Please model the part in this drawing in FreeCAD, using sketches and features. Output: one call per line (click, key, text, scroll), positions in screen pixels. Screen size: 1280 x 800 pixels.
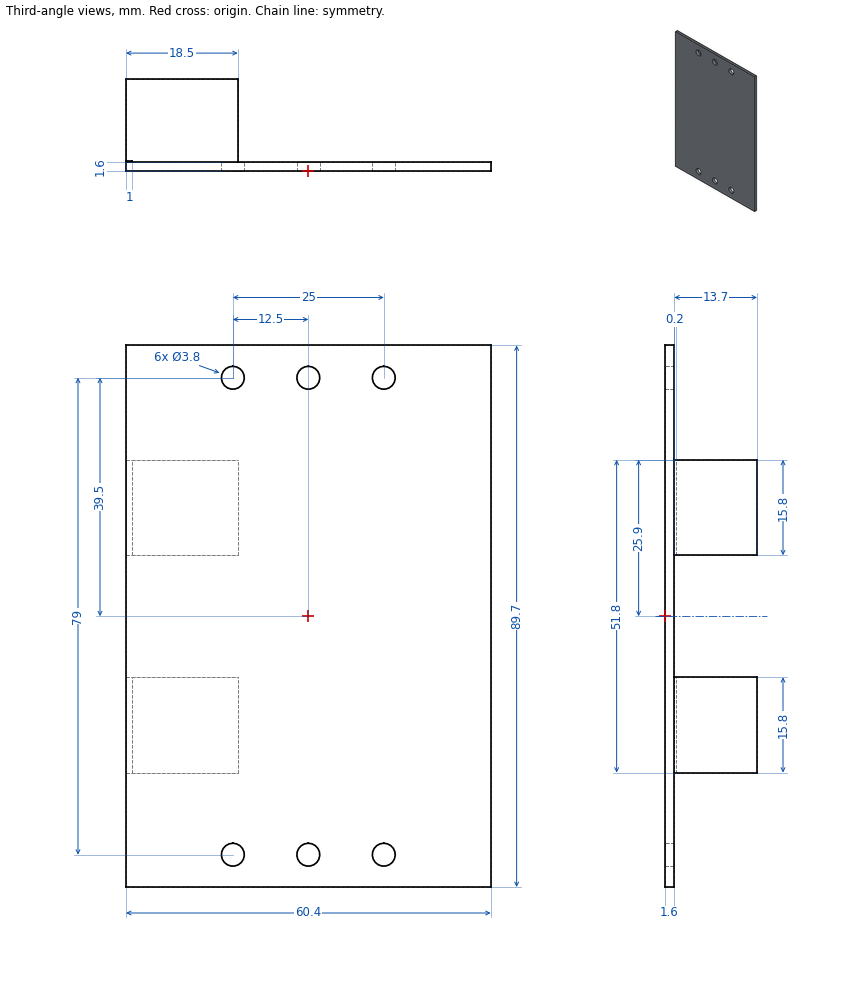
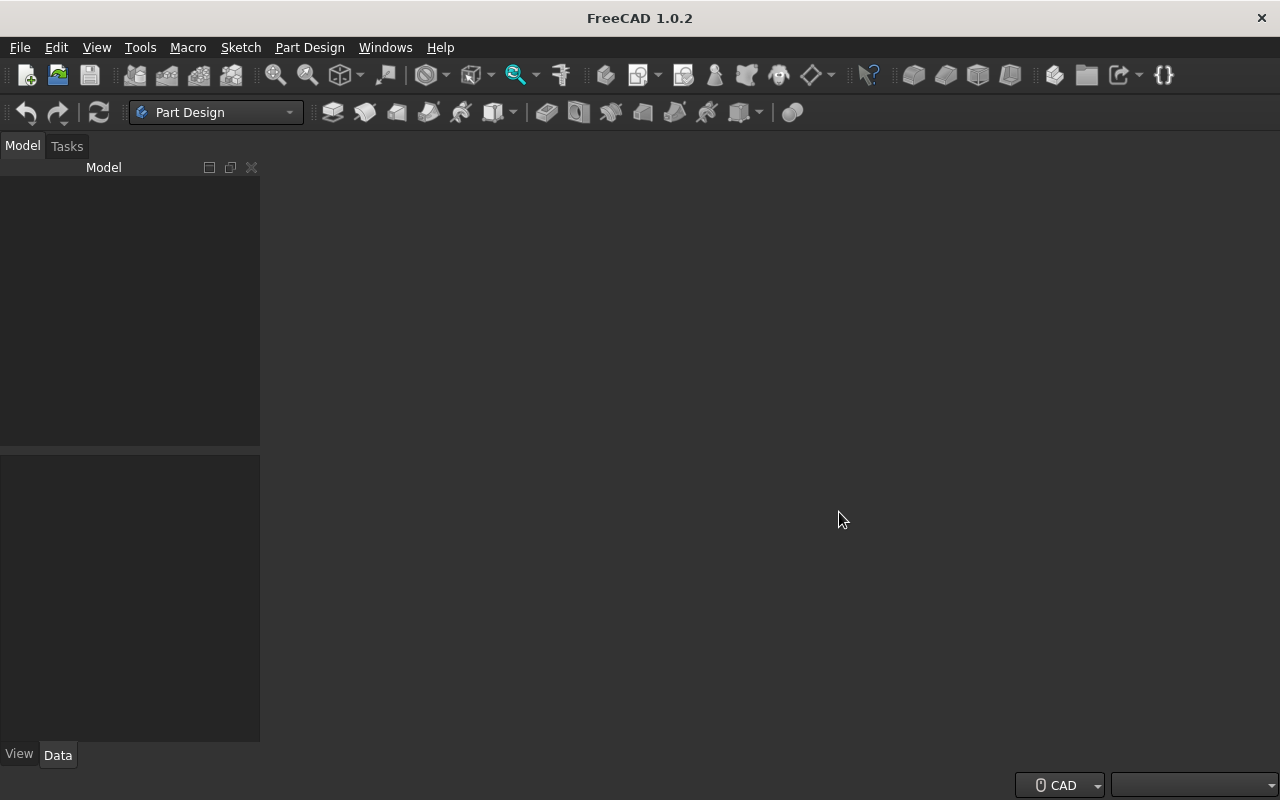
click(26, 76)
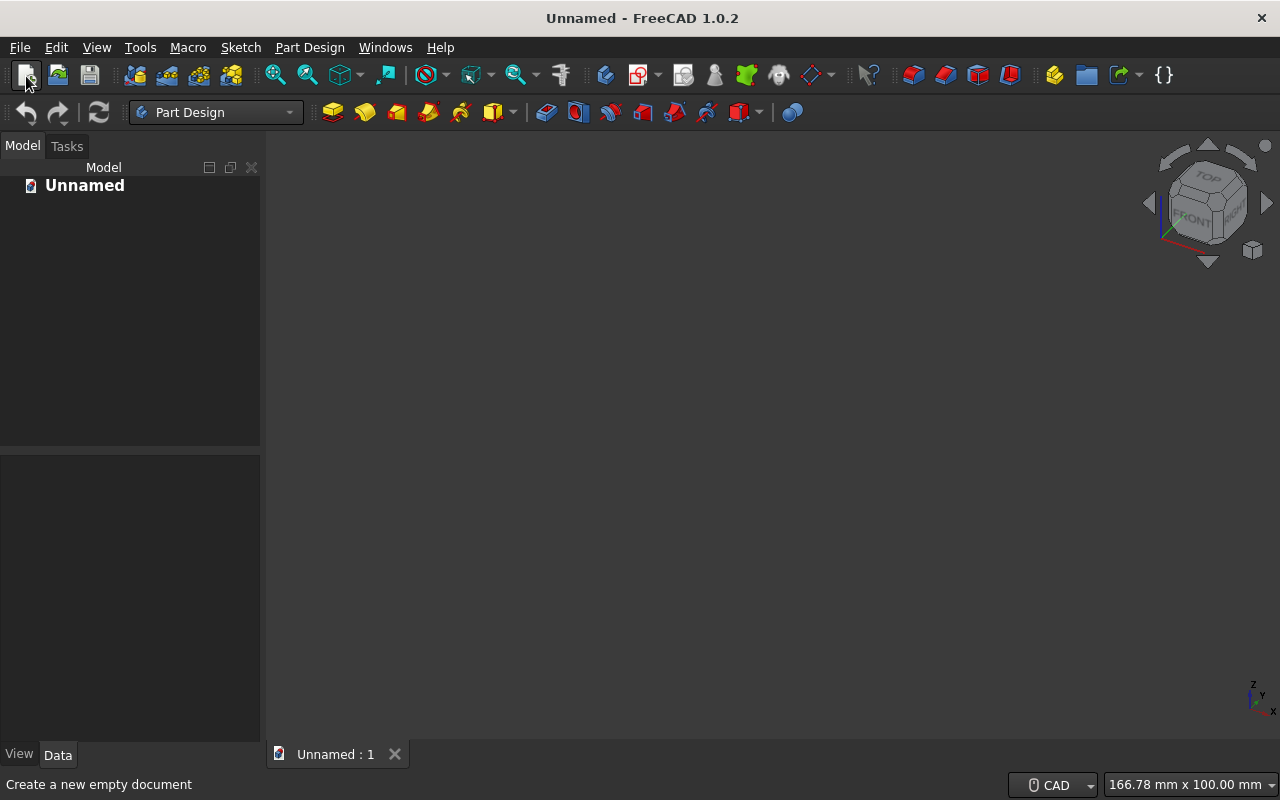
click(638, 76)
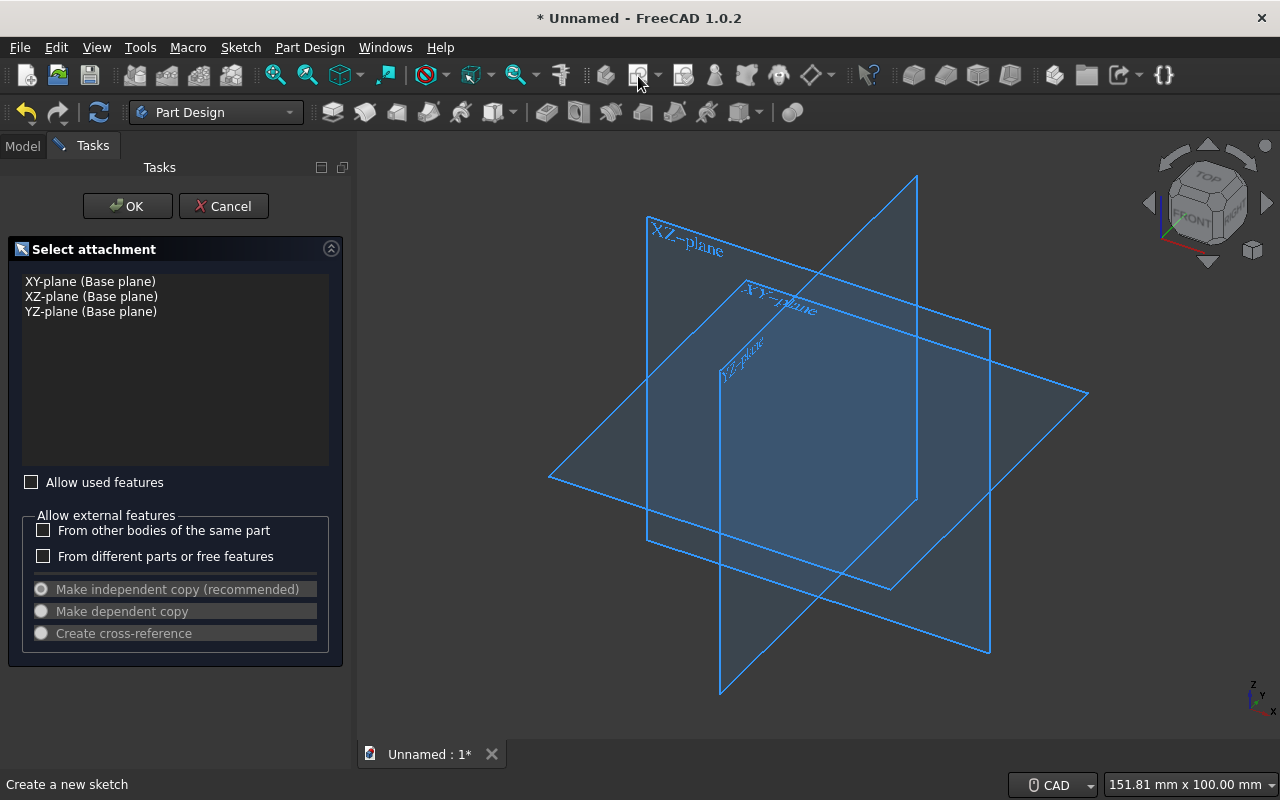
click(82, 296)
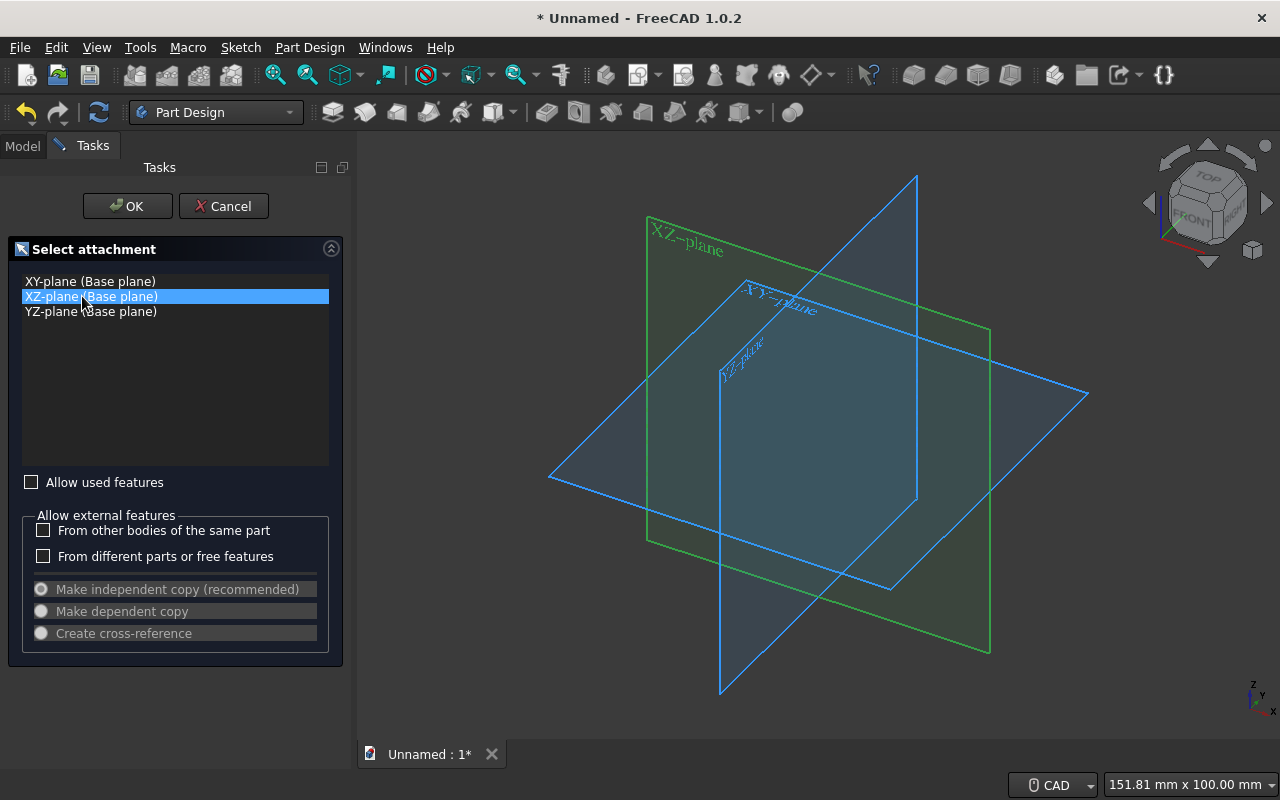
click(128, 206)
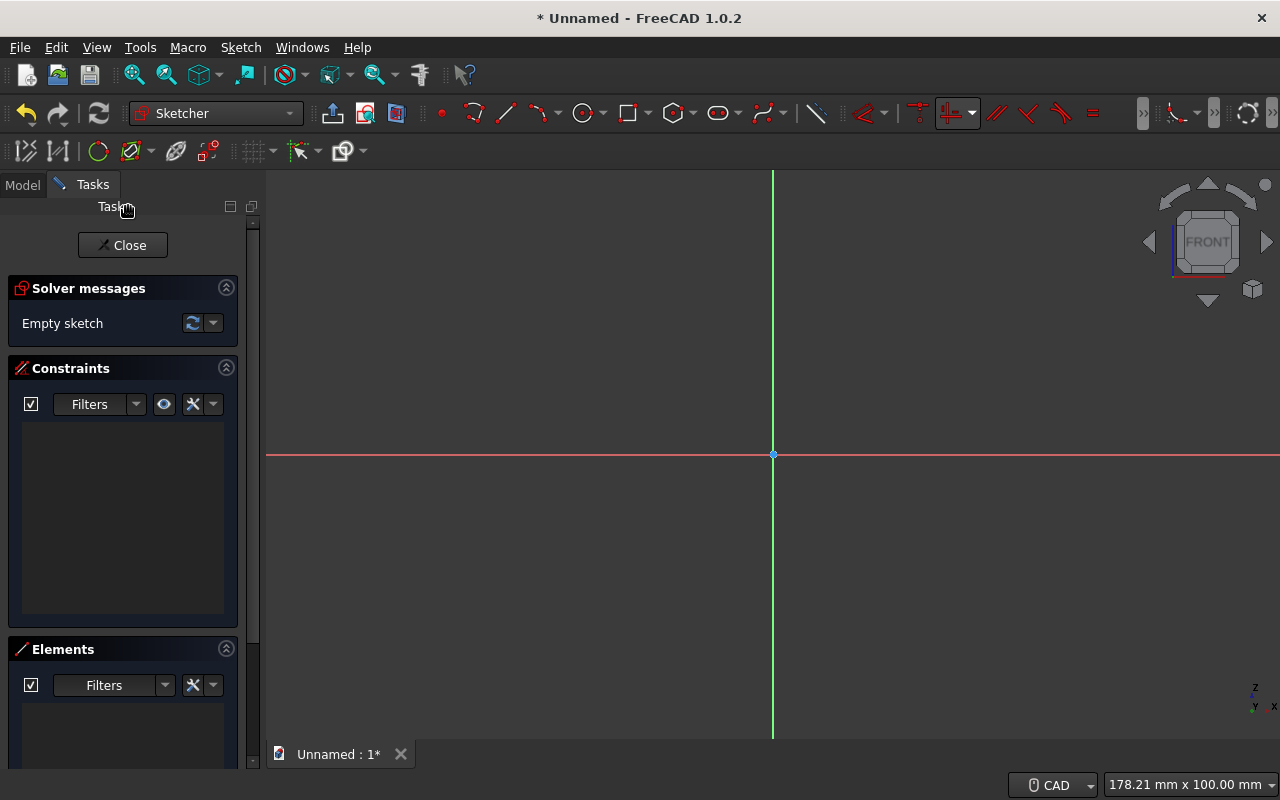
scroll(565, 455, down, 2)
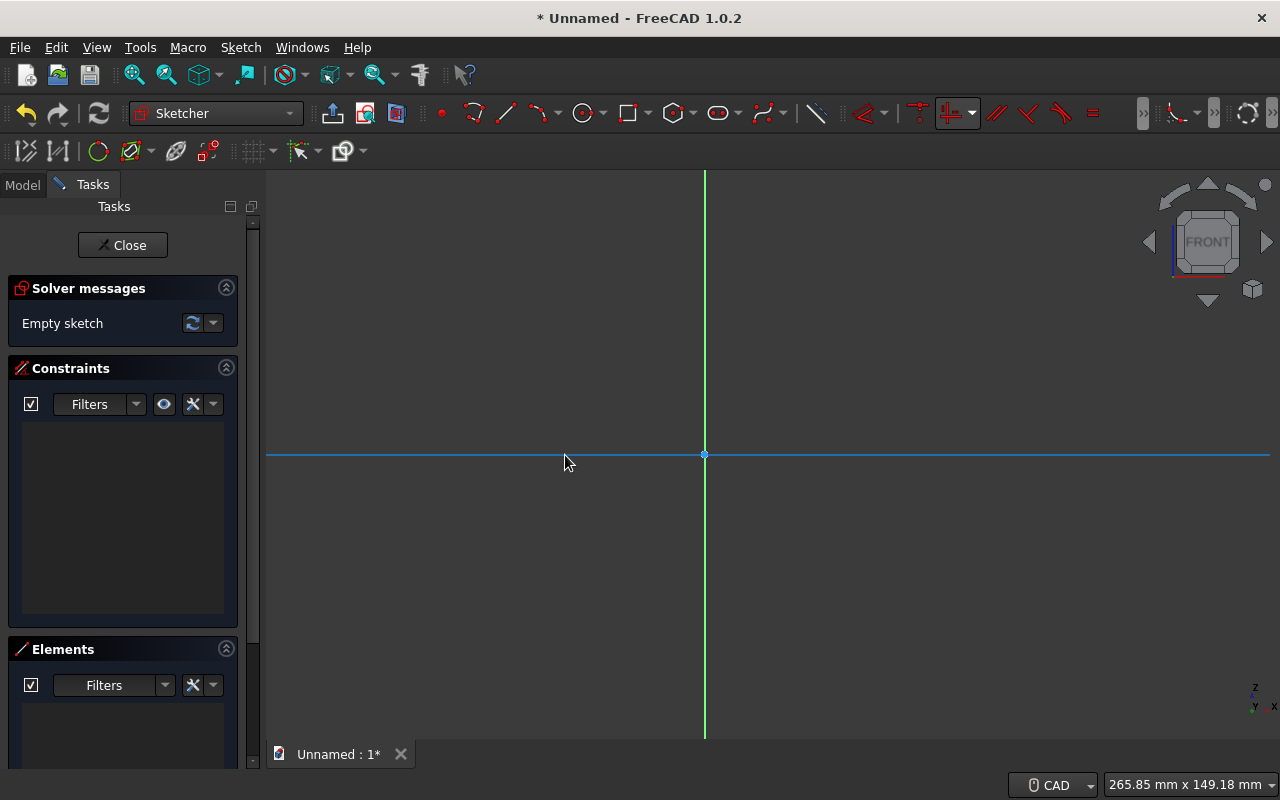
key(g)
key(v)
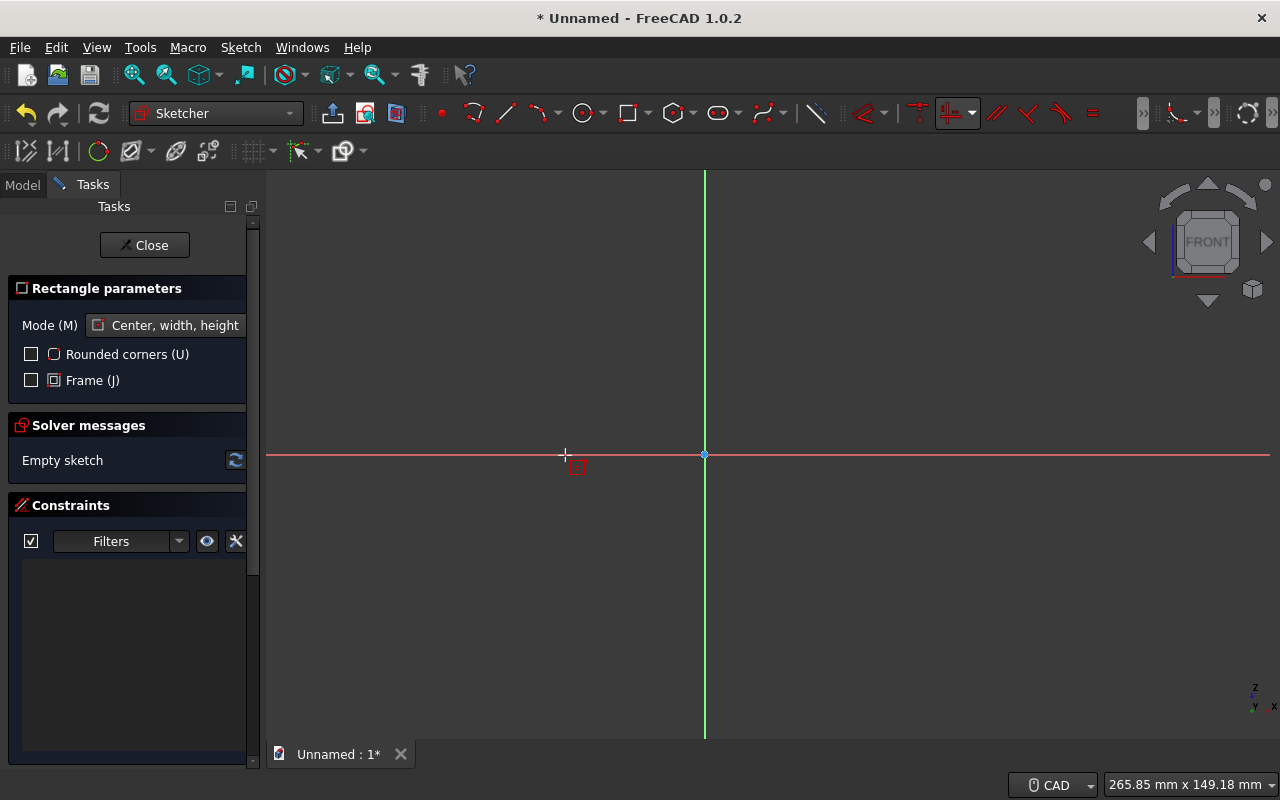
click(705, 455)
move(820, 284)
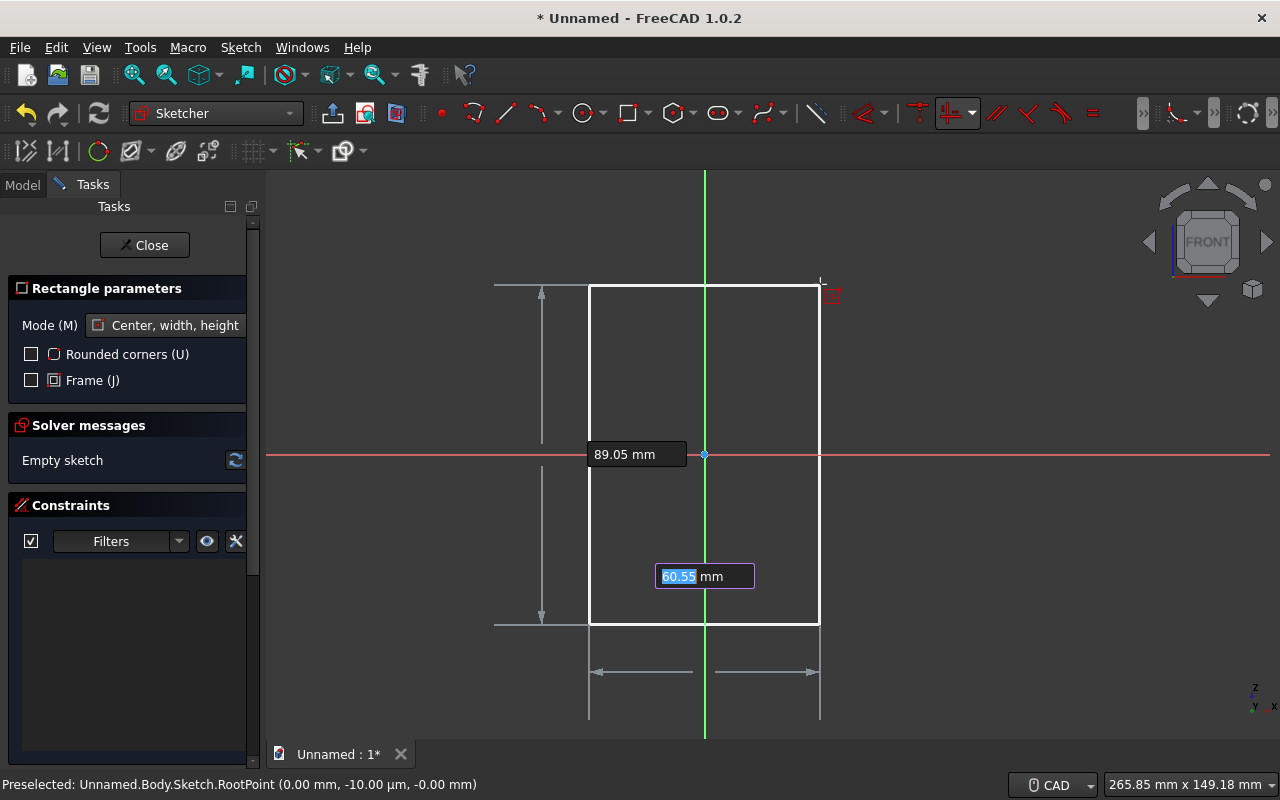
text(60.4)
key(Tab)
text(89.7)
key(Return)
key(Escape)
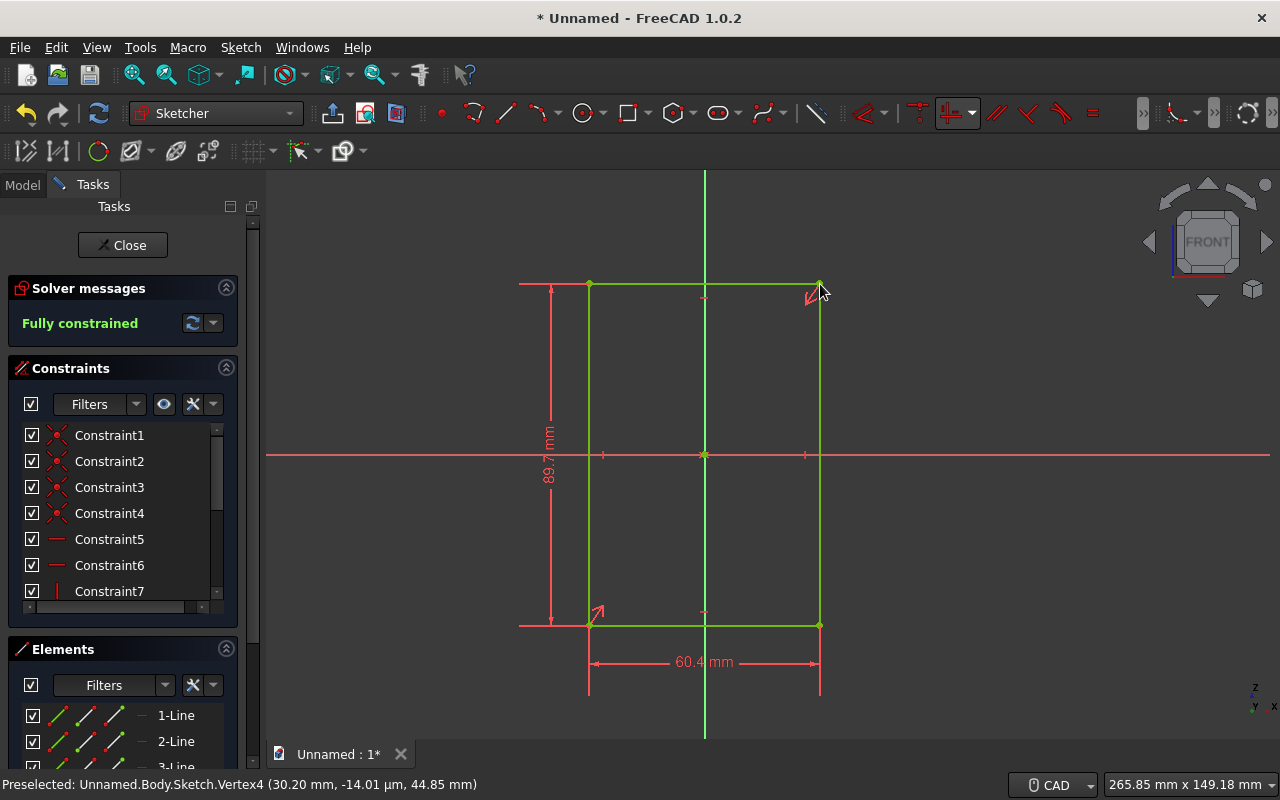
click(123, 245)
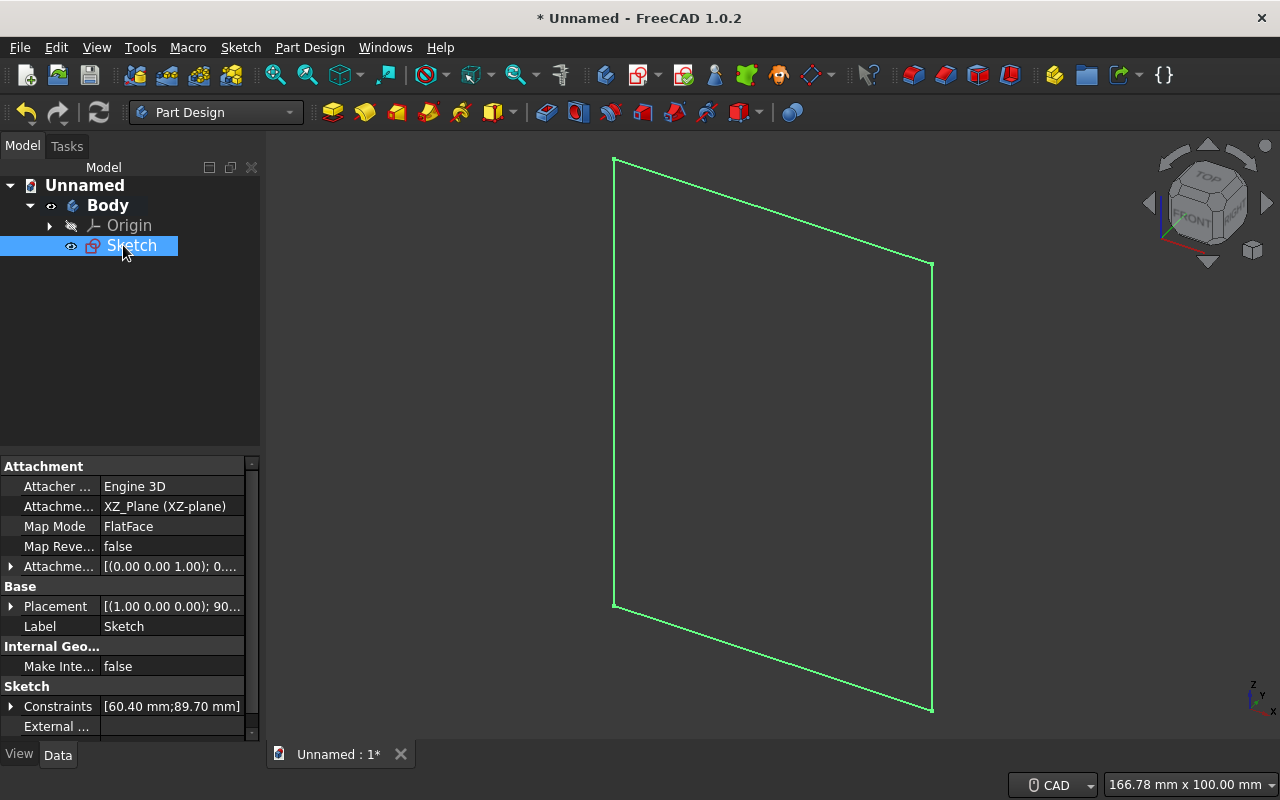
click(334, 112)